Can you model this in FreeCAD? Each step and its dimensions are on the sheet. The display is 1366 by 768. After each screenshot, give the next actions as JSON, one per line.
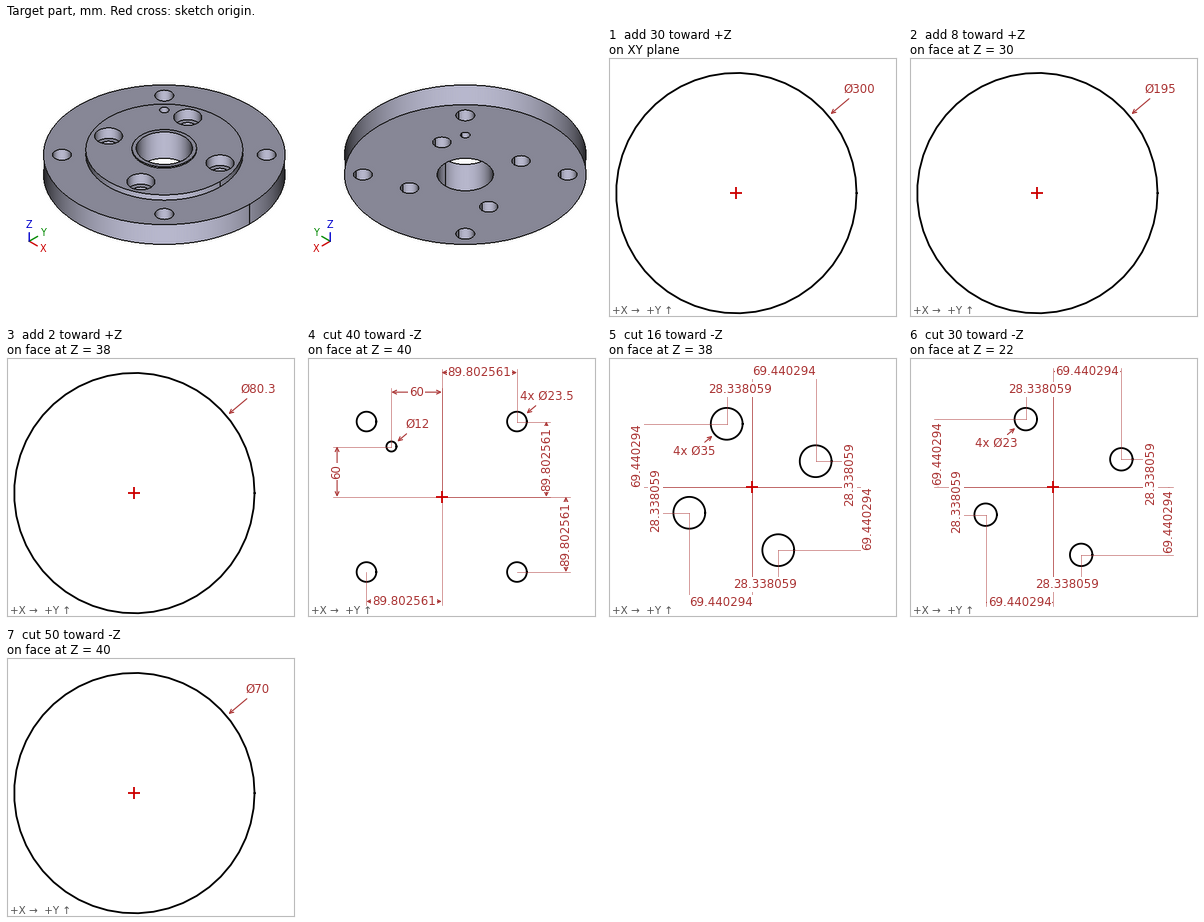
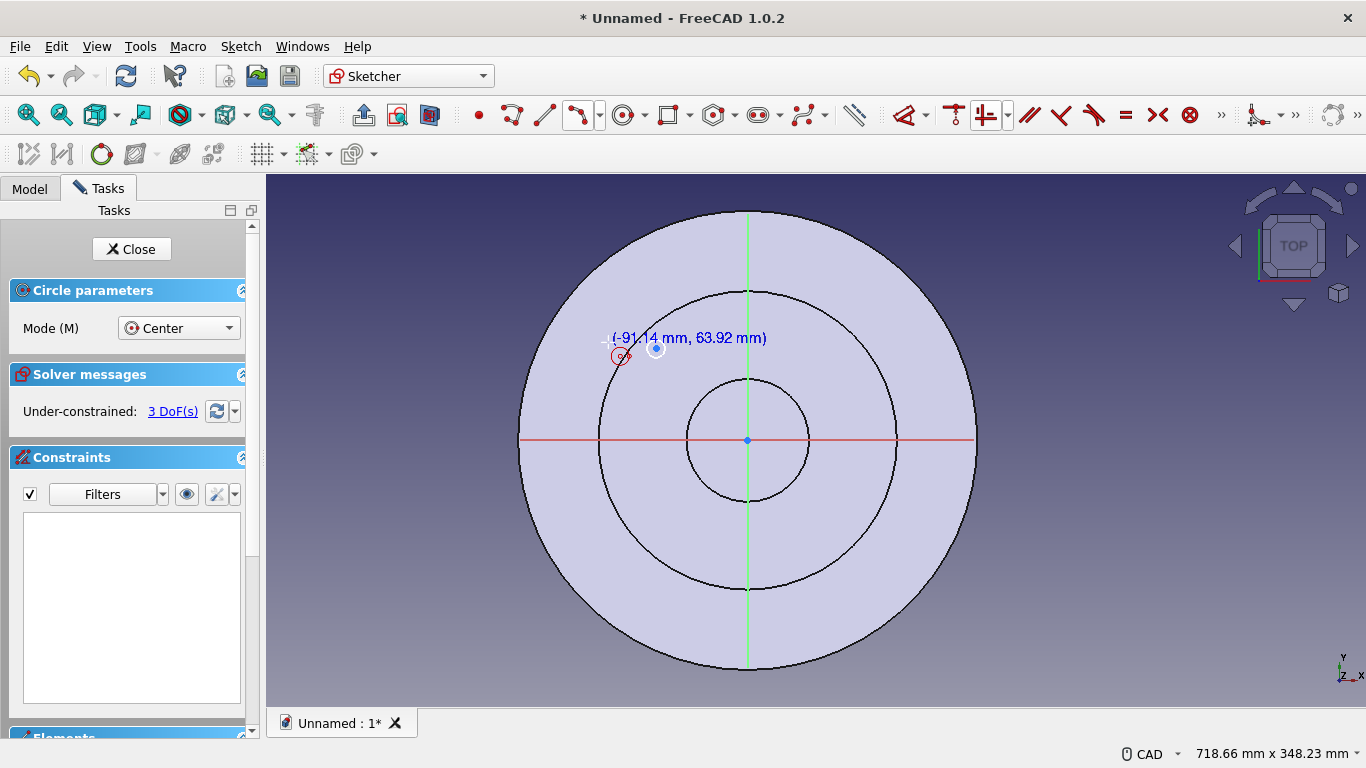
{"action": "scroll", "coordinate": [885, 303], "scroll_direction": "up", "scroll_amount": 2}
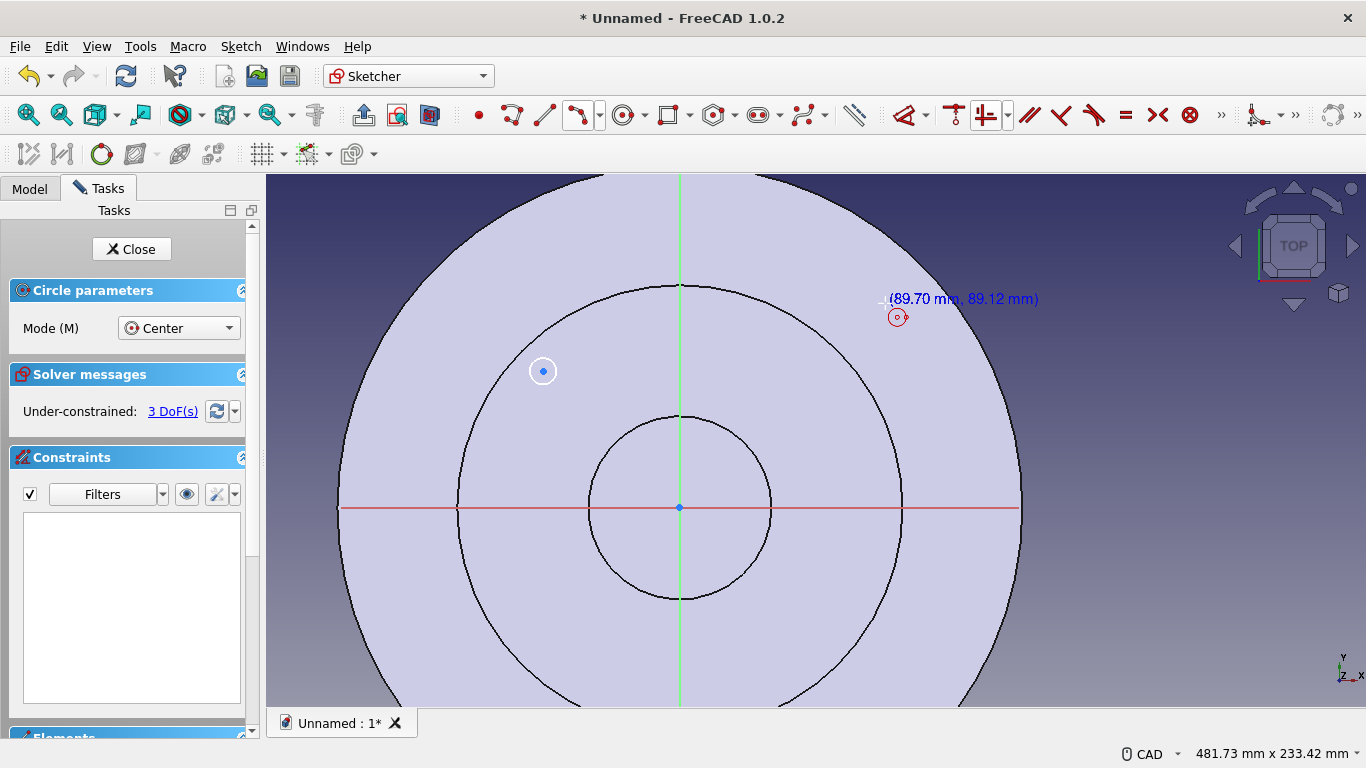
{"action": "left_click", "coordinate": [885, 303]}
{"action": "left_click", "coordinate": [904, 284]}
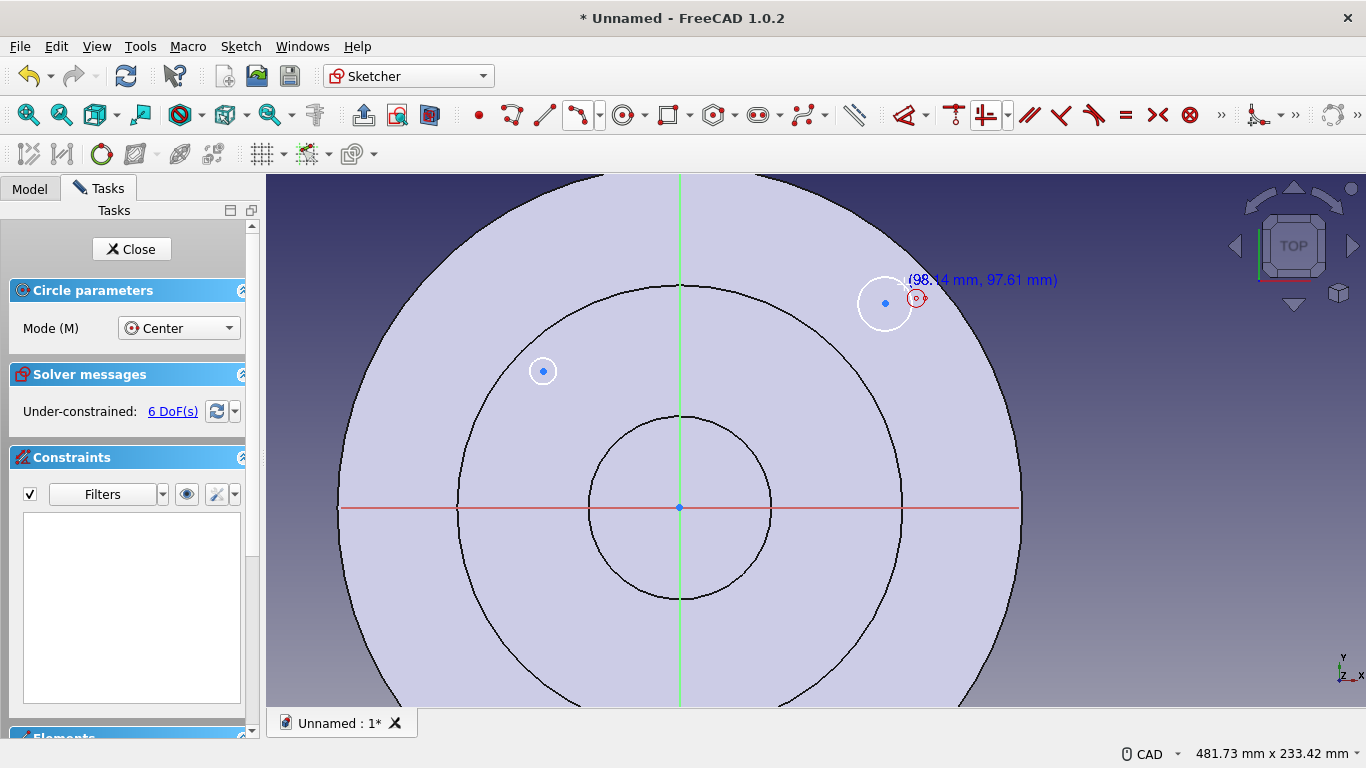
{"action": "scroll", "coordinate": [885, 304], "scroll_direction": "down", "scroll_amount": 2}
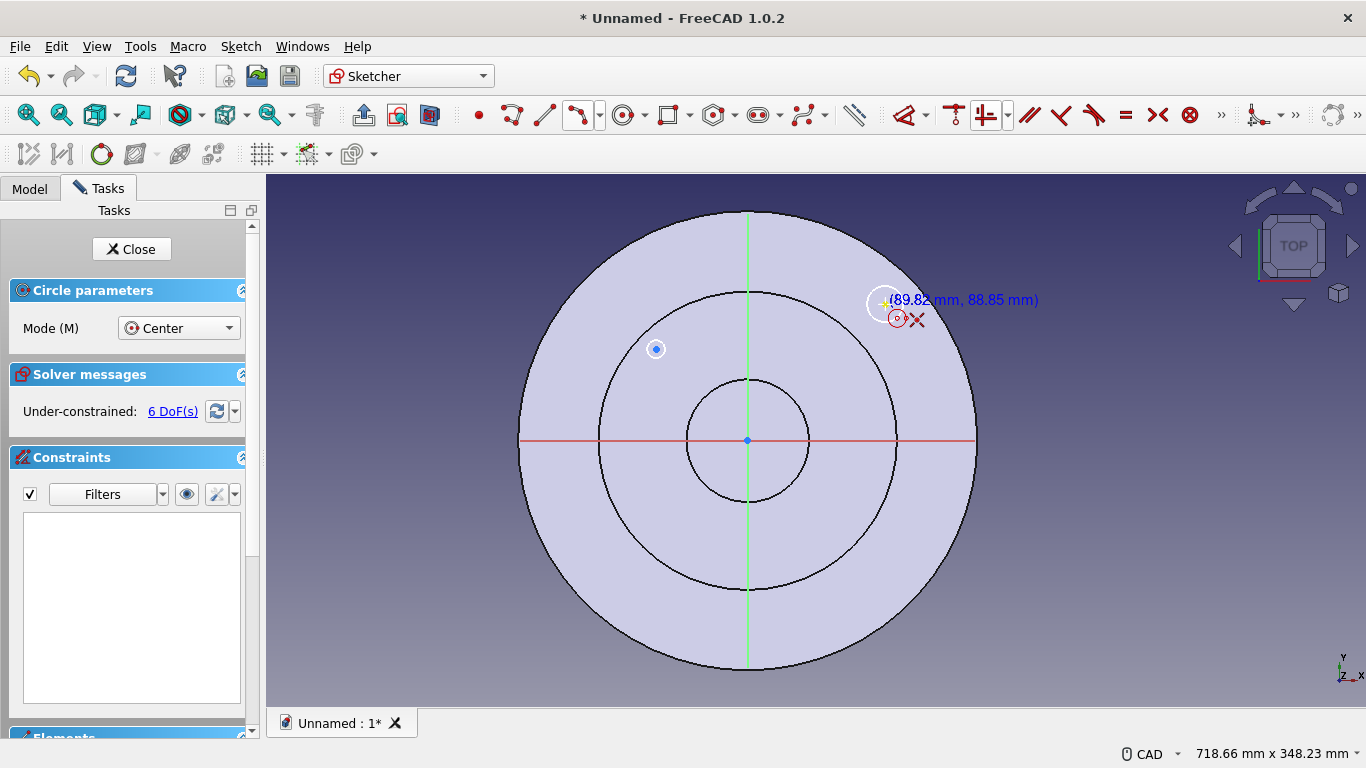
{"action": "scroll", "coordinate": [885, 578], "scroll_direction": "up", "scroll_amount": 2}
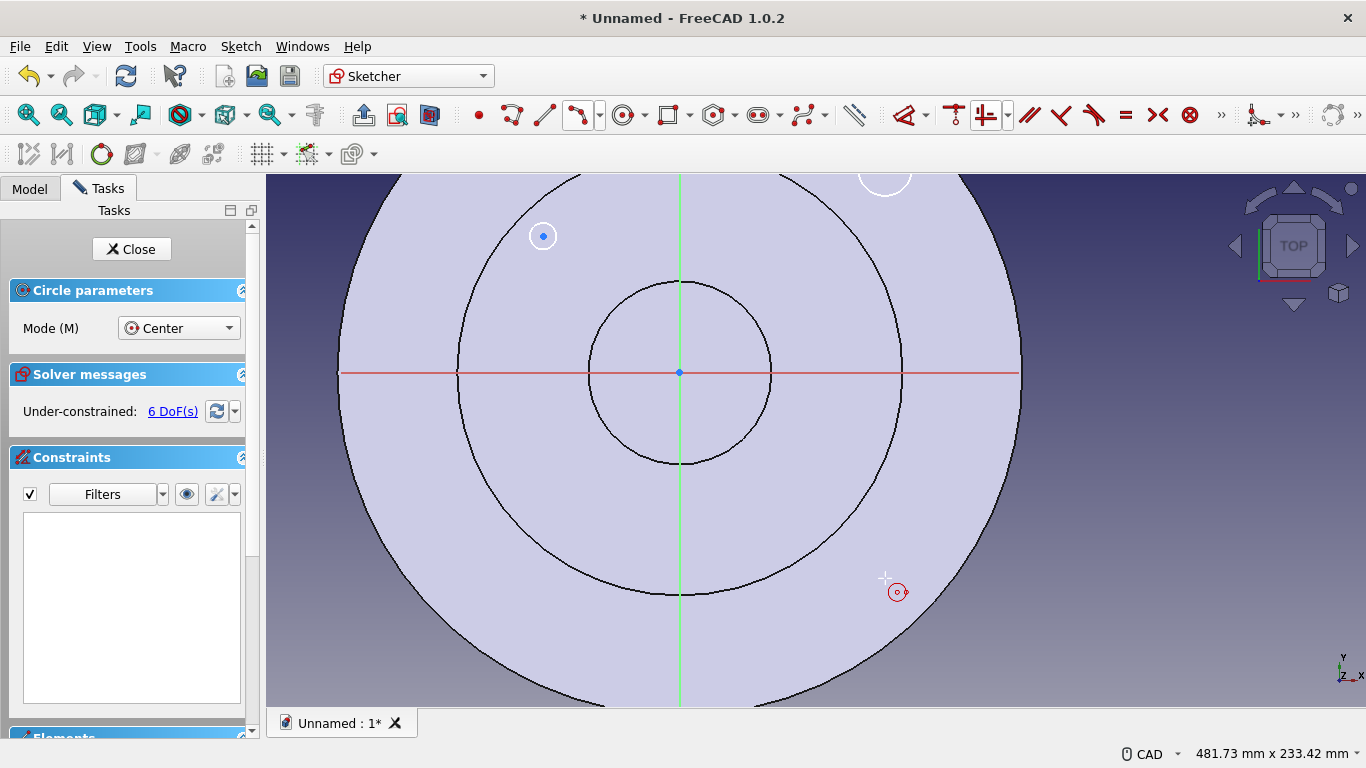
{"action": "left_click", "coordinate": [885, 578]}
{"action": "left_click", "coordinate": [904, 559]}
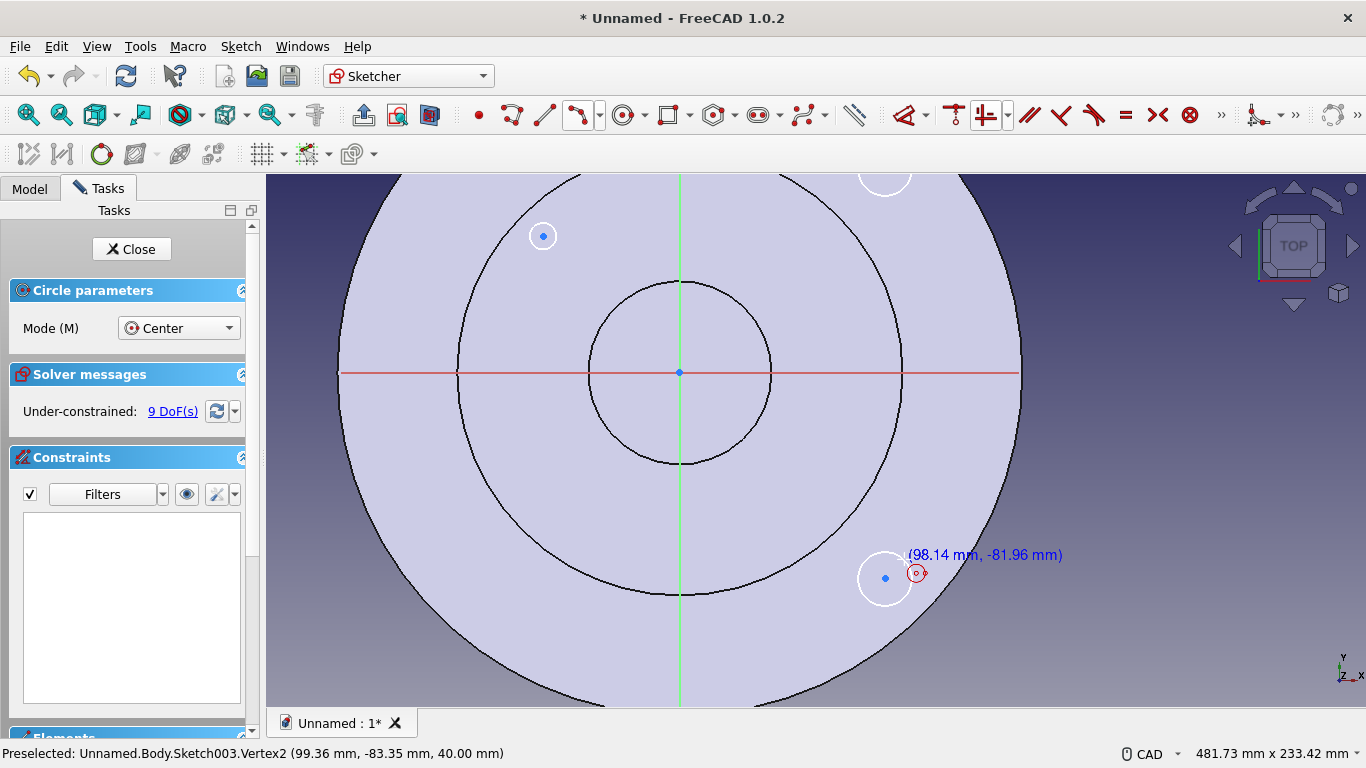
{"action": "left_click", "coordinate": [475, 578]}
{"action": "left_click", "coordinate": [494, 559]}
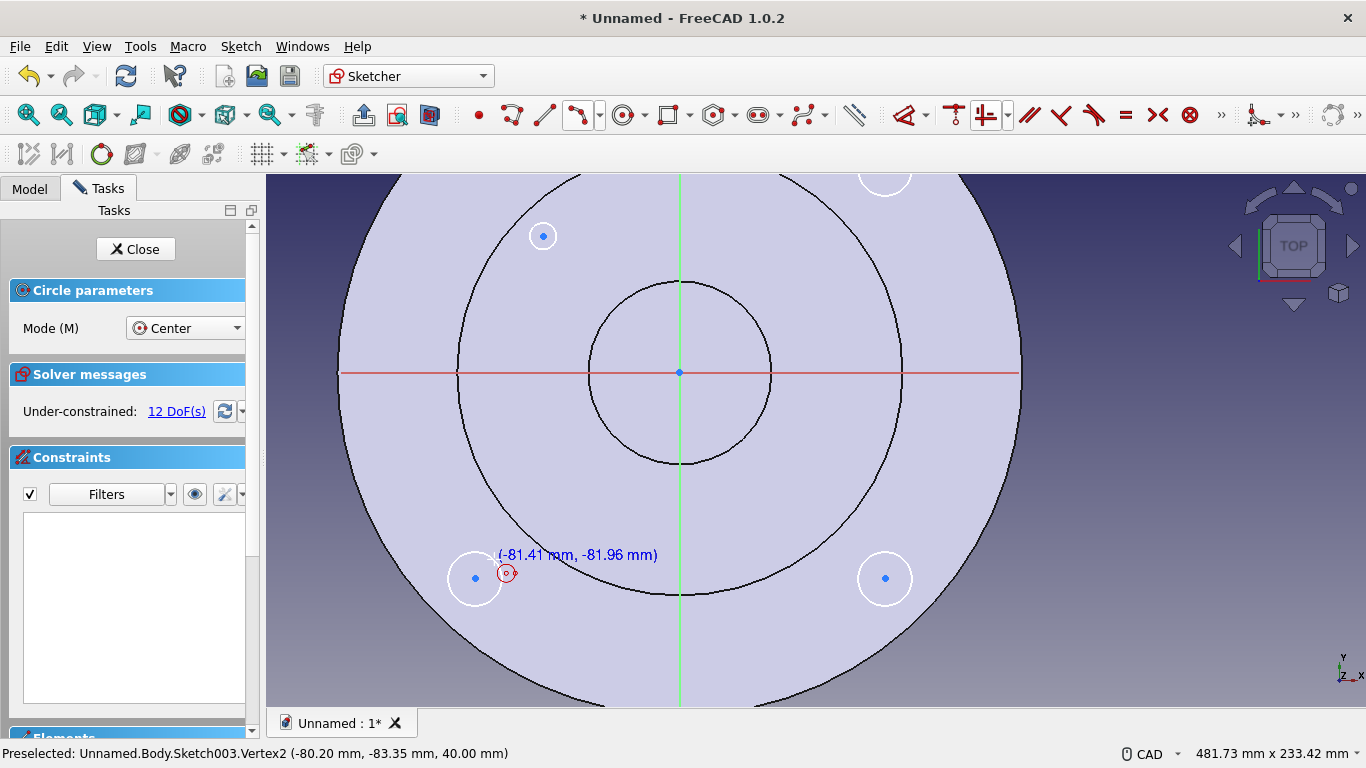
{"action": "scroll", "coordinate": [885, 578], "scroll_direction": "down", "scroll_amount": 2}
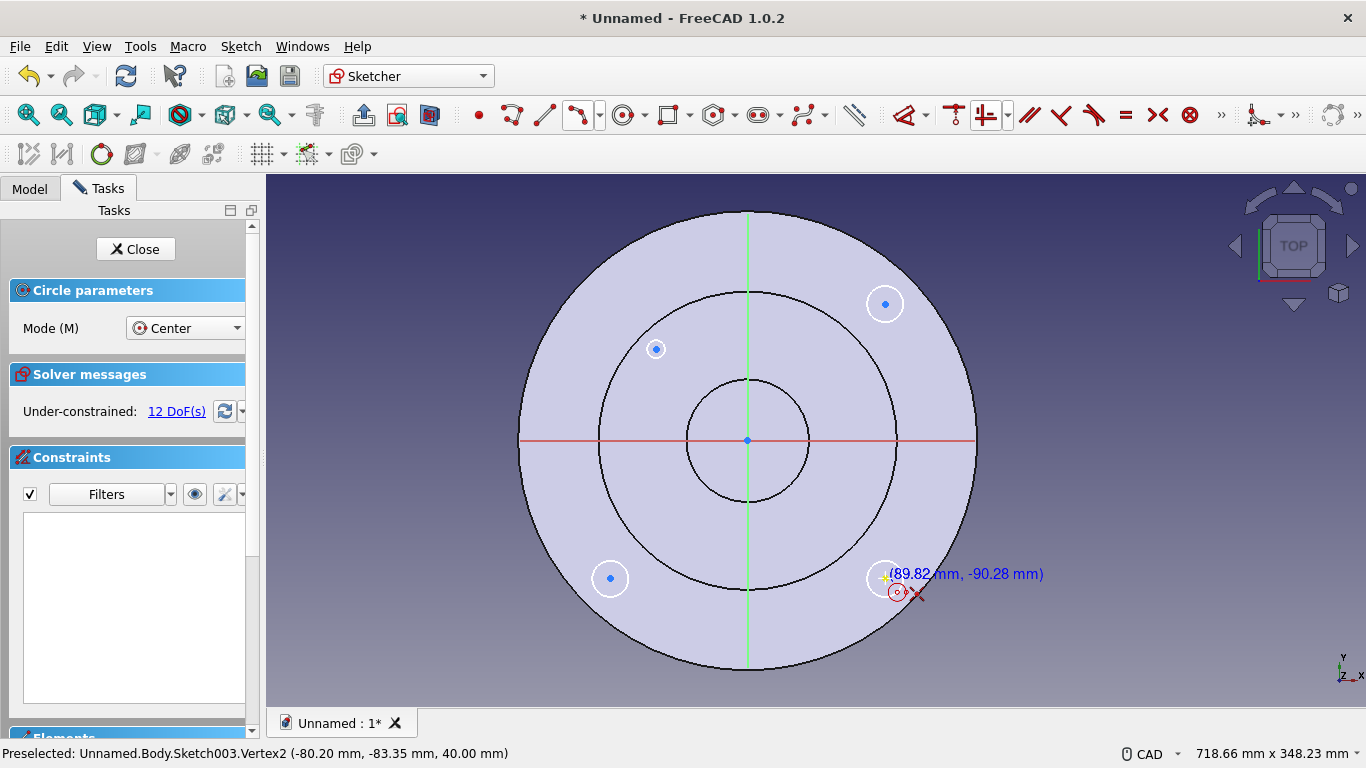
{"action": "scroll", "coordinate": [610, 303], "scroll_direction": "up", "scroll_amount": 2}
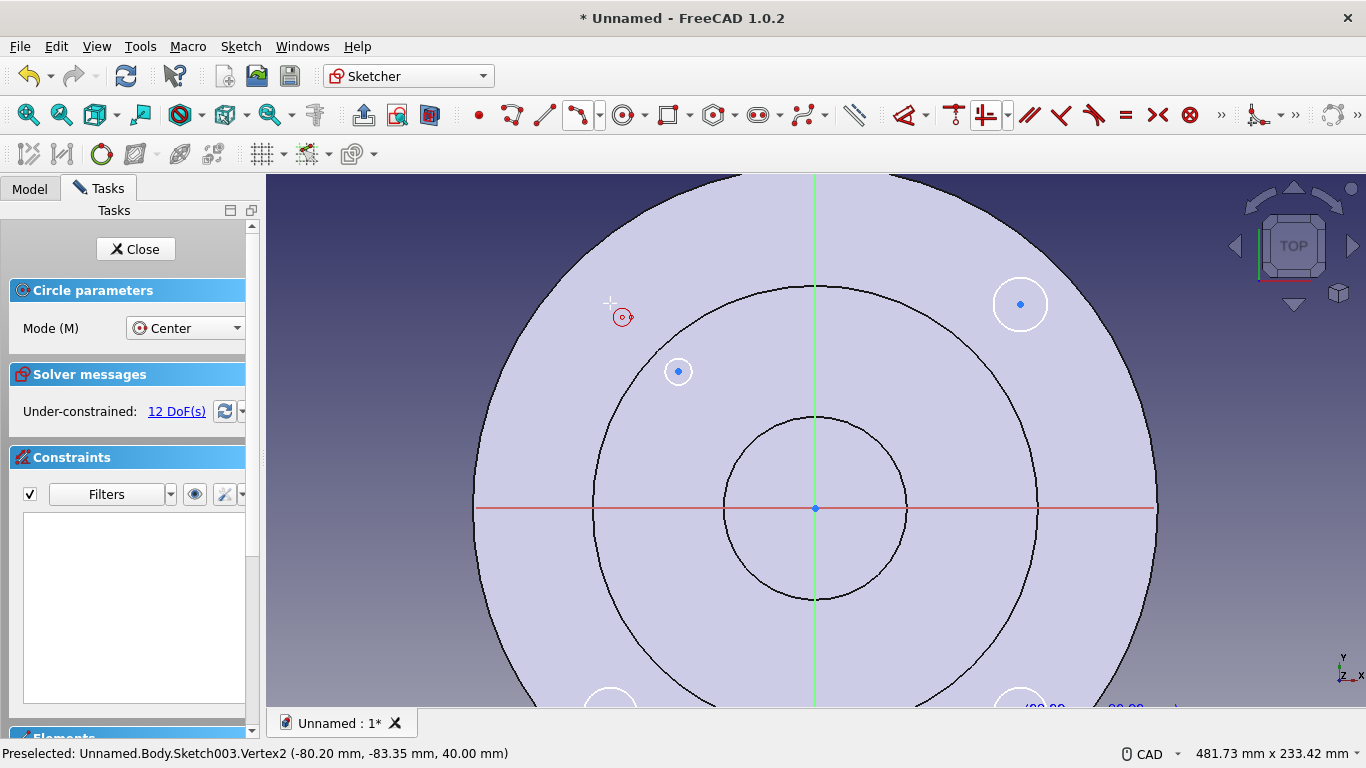
{"action": "left_click", "coordinate": [610, 303]}
{"action": "left_click", "coordinate": [629, 284]}
{"action": "key", "text": "Escape"}